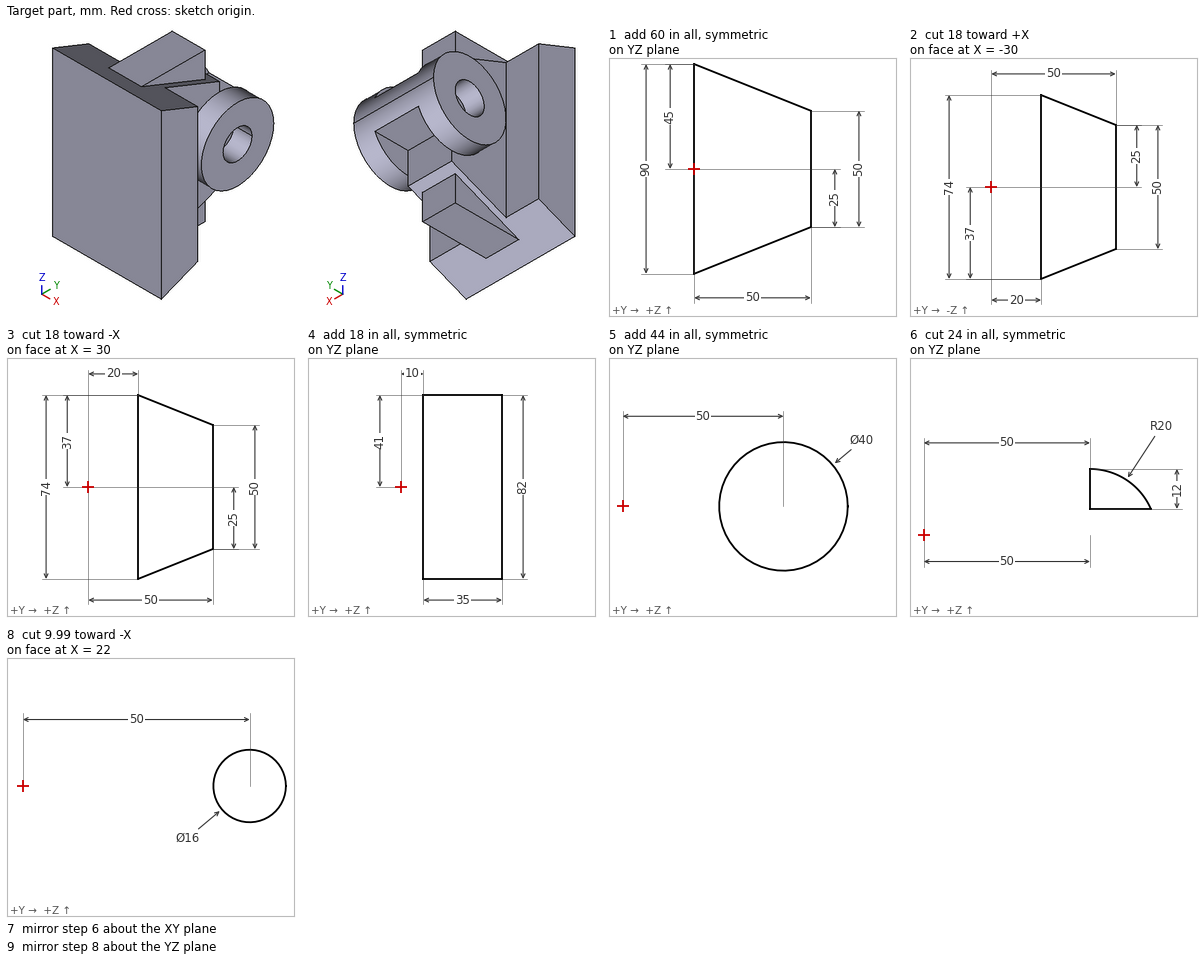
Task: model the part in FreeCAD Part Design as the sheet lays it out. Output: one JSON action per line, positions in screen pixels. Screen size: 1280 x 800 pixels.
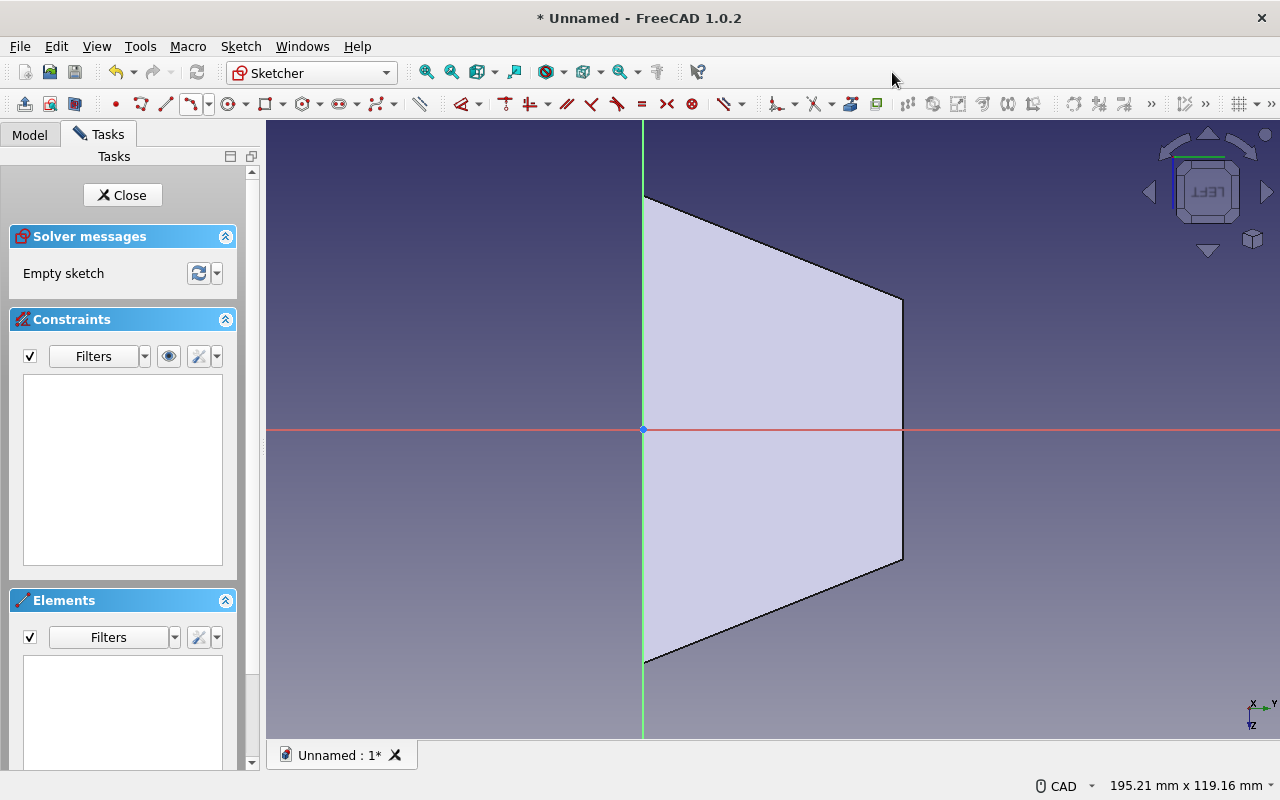
{"action": "left_click", "coordinate": [747, 622]}
{"action": "left_click", "coordinate": [747, 237]}
{"action": "left_click", "coordinate": [903, 300]}
{"action": "left_click", "coordinate": [903, 559]}
{"action": "left_click", "coordinate": [747, 623]}
{"action": "key", "text": "Escape"}
{"action": "key", "text": "Escape"}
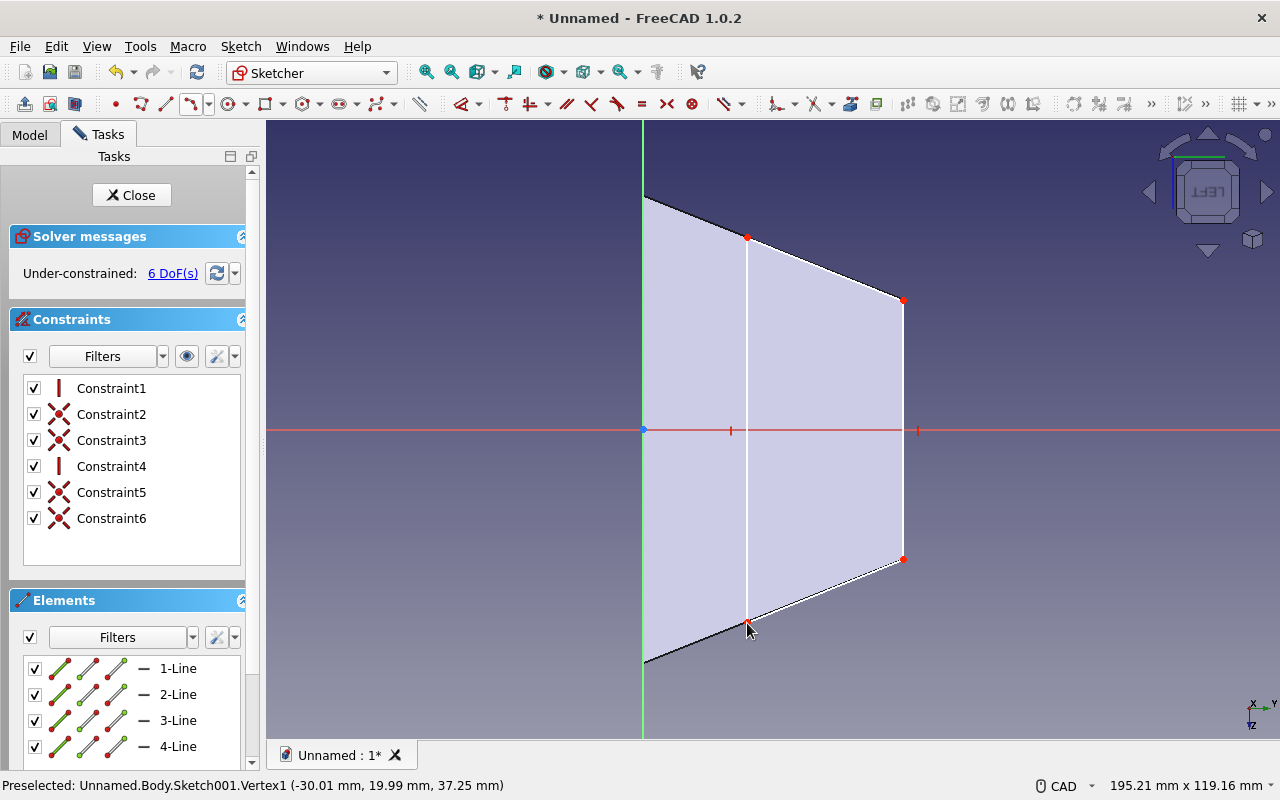
{"action": "left_click", "coordinate": [460, 104]}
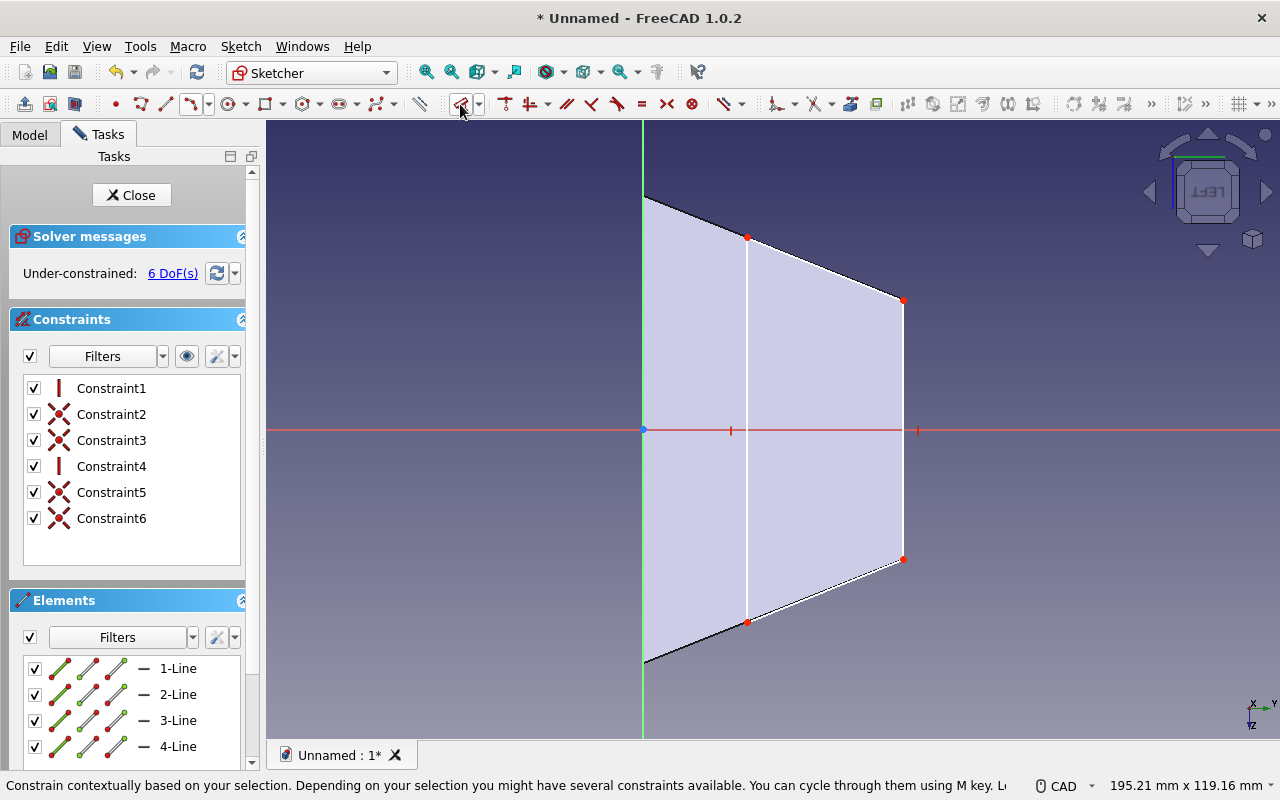
{"action": "left_click", "coordinate": [747, 507]}
{"action": "left_click", "coordinate": [713, 342]}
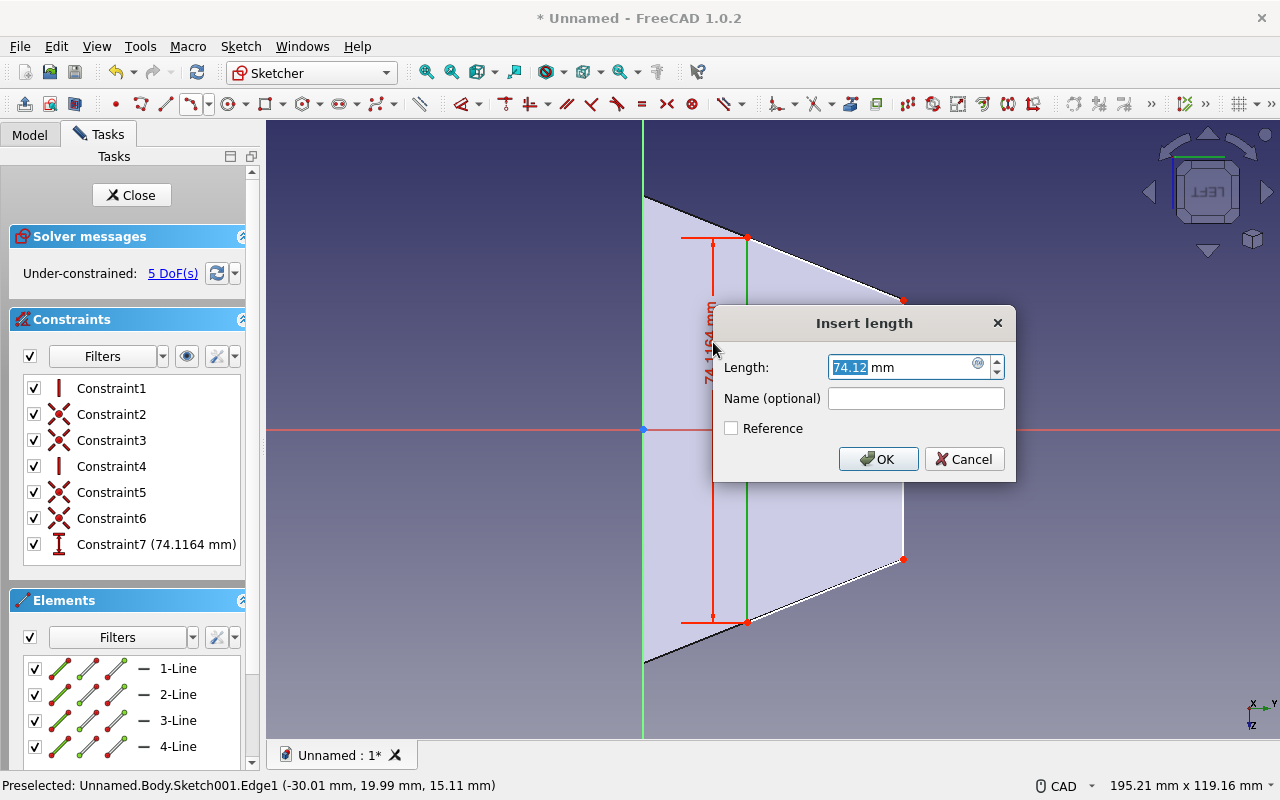
{"action": "type", "text": "74"}
{"action": "key", "text": "Return"}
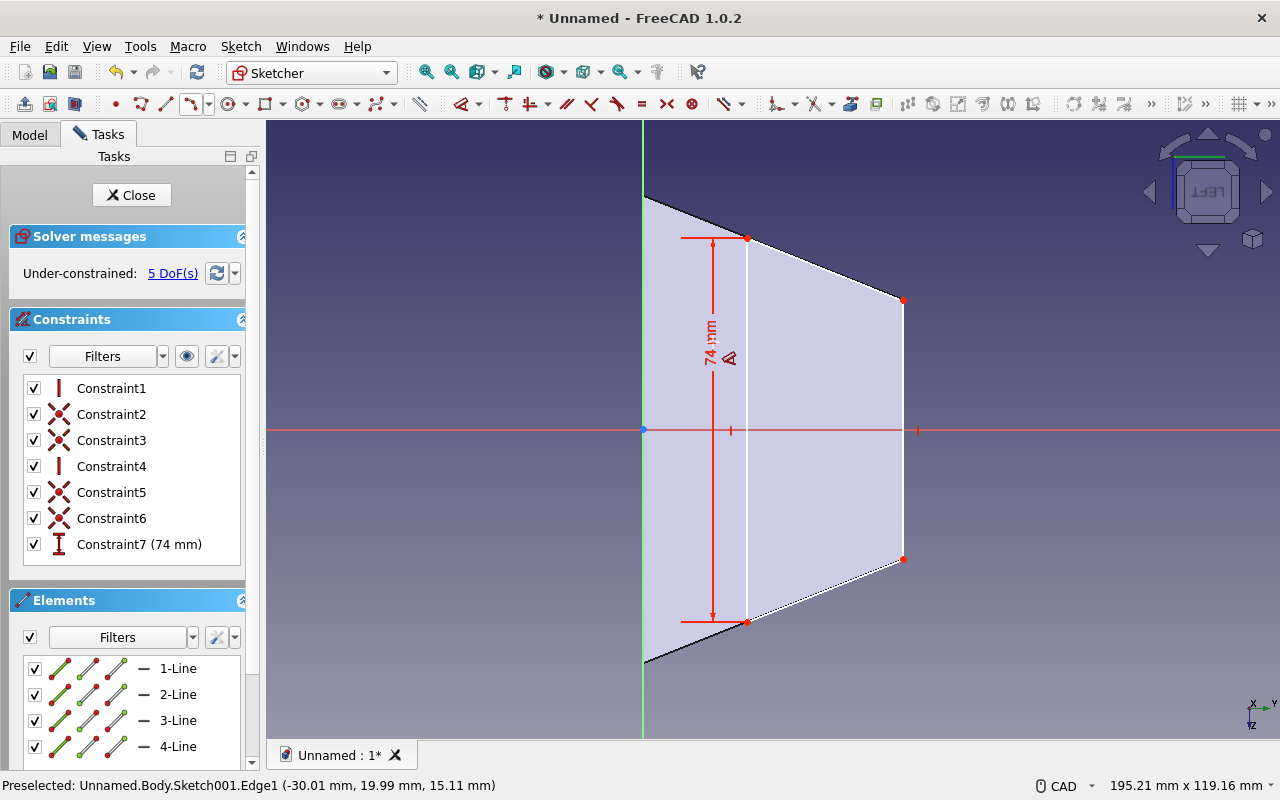
{"action": "left_click", "coordinate": [903, 379]}
{"action": "left_click", "coordinate": [937, 371]}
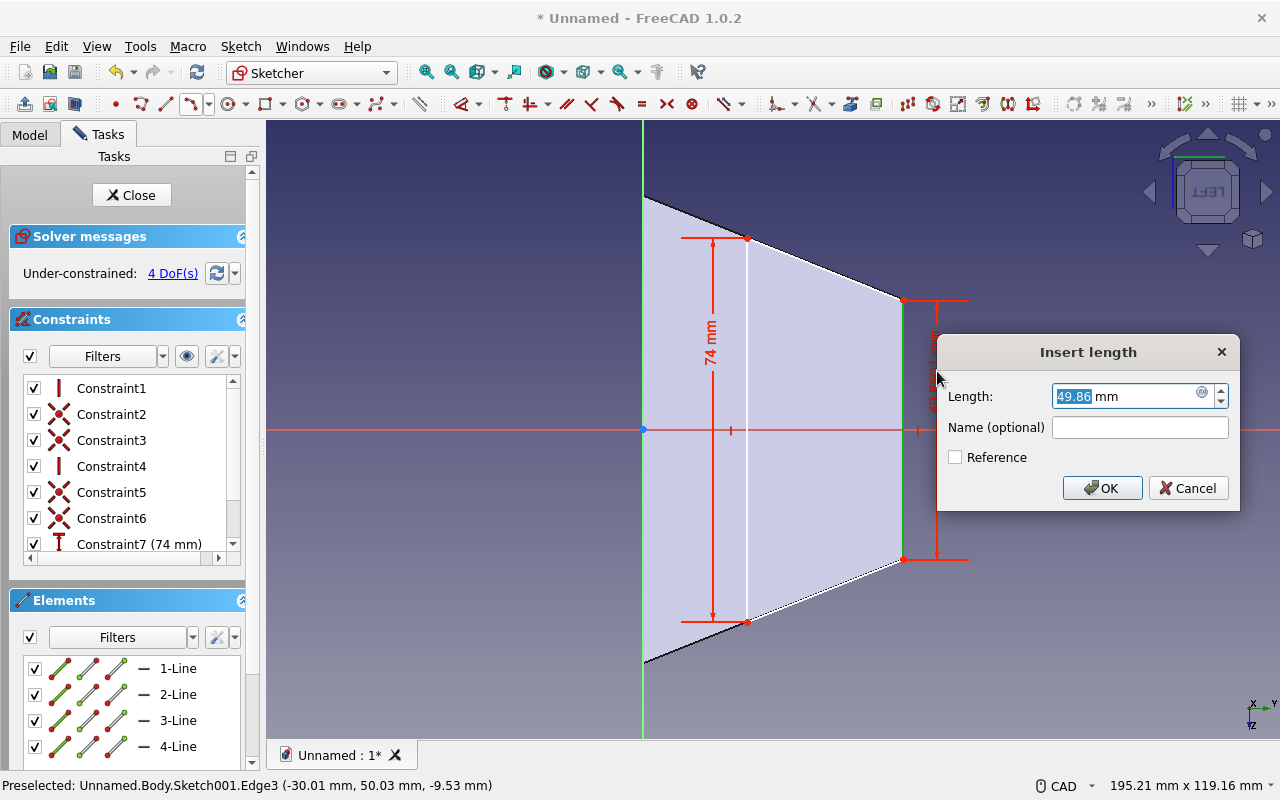
{"action": "type", "text": "50"}
{"action": "key", "text": "Return"}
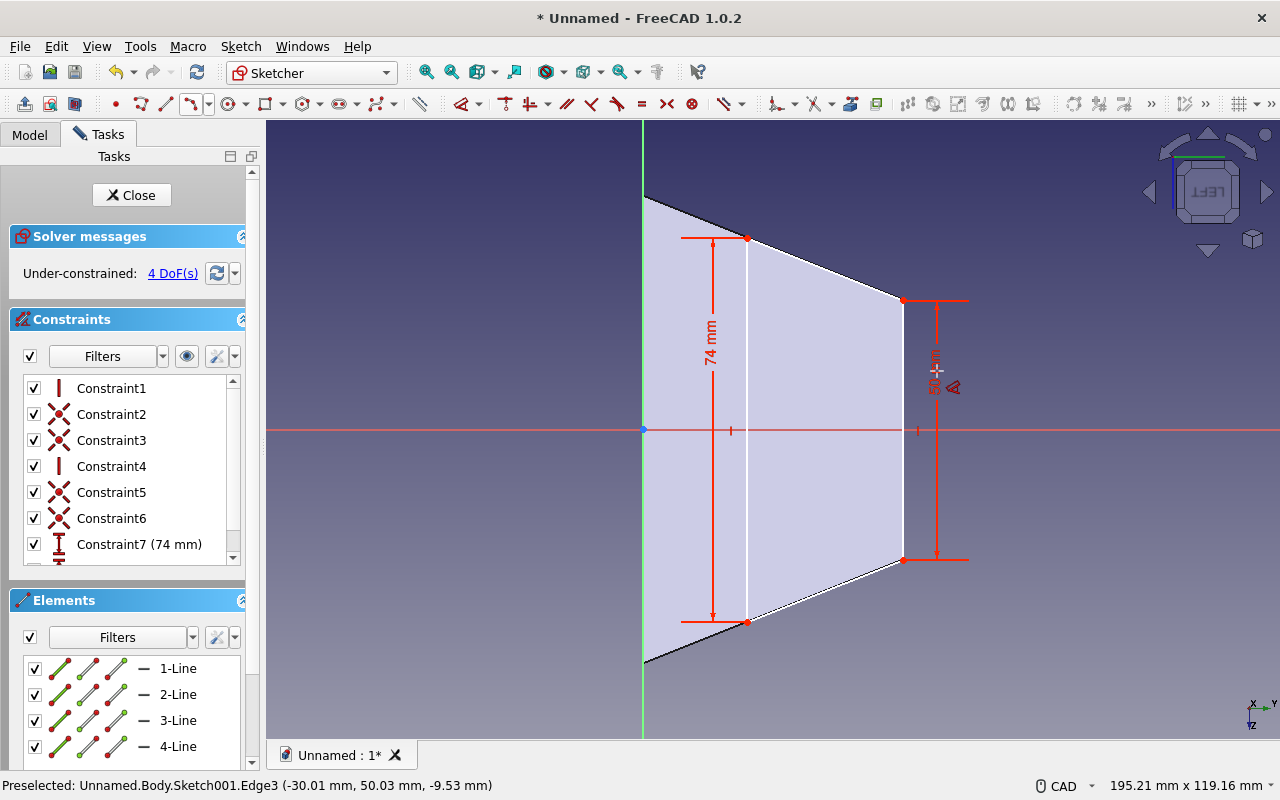
{"action": "left_click", "coordinate": [747, 622]}
{"action": "left_click", "coordinate": [695, 656]}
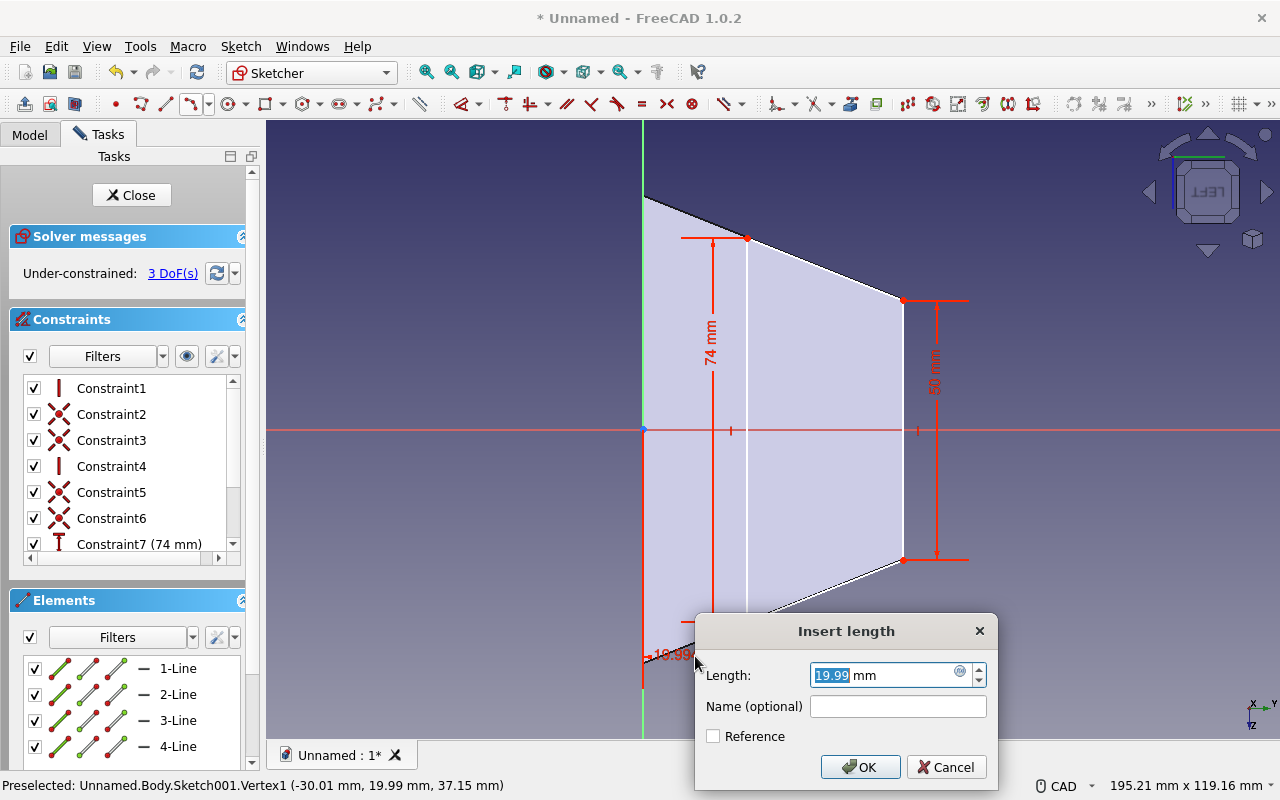
{"action": "type", "text": "20"}
{"action": "key", "text": "Return"}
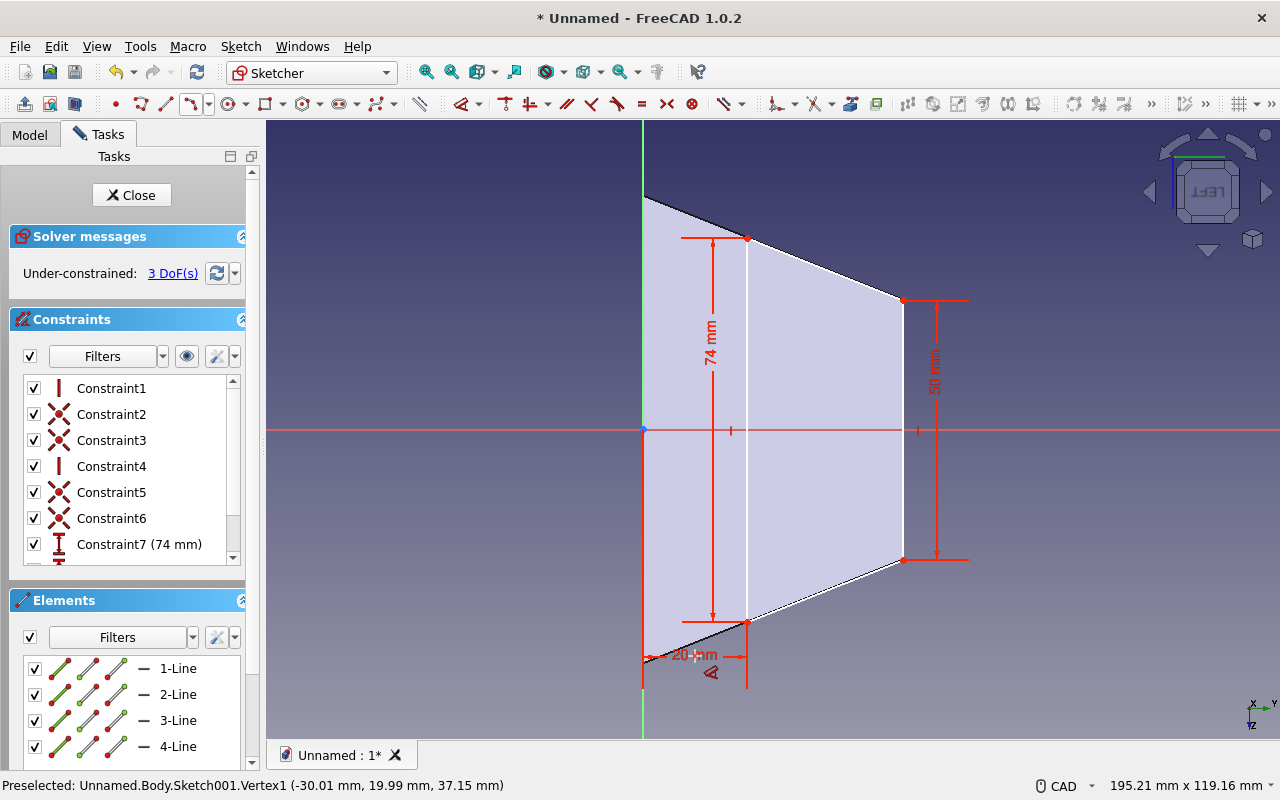
{"action": "left_click", "coordinate": [747, 622]}
{"action": "left_click", "coordinate": [609, 526]}